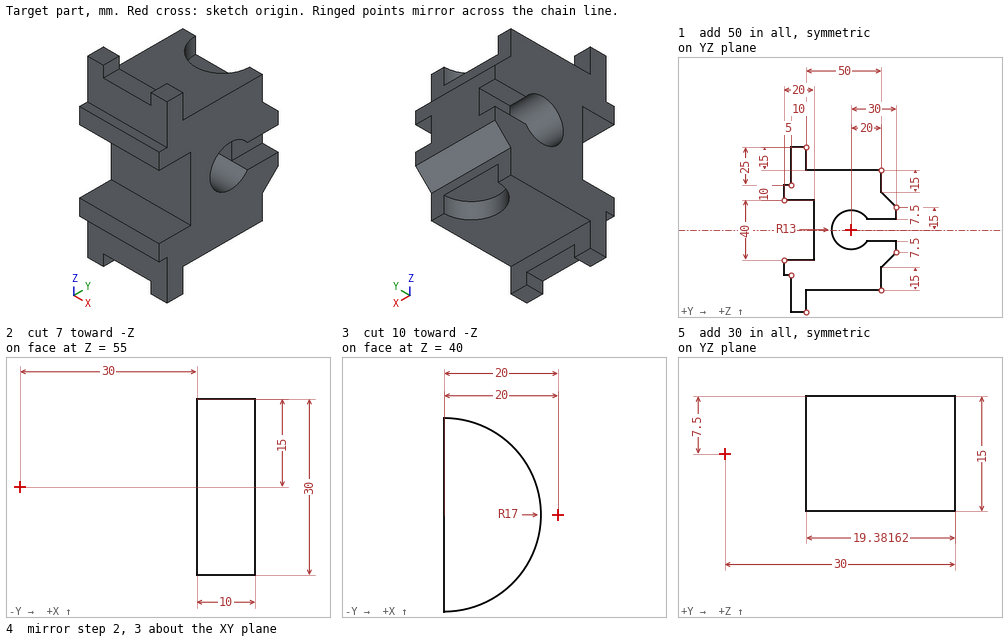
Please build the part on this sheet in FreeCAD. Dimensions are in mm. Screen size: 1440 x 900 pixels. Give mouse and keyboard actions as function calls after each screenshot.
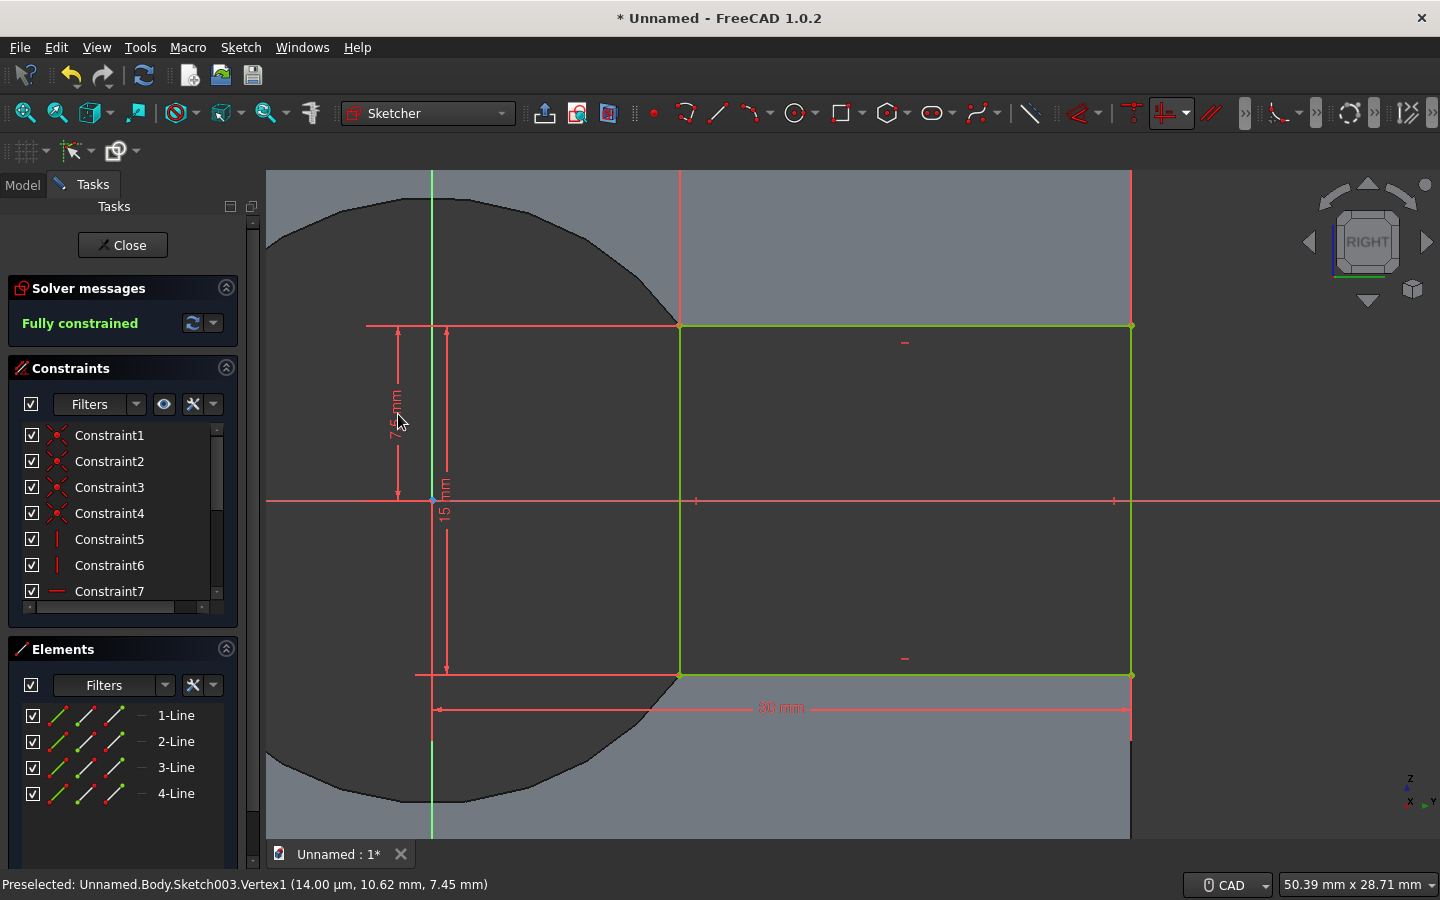
click(123, 245)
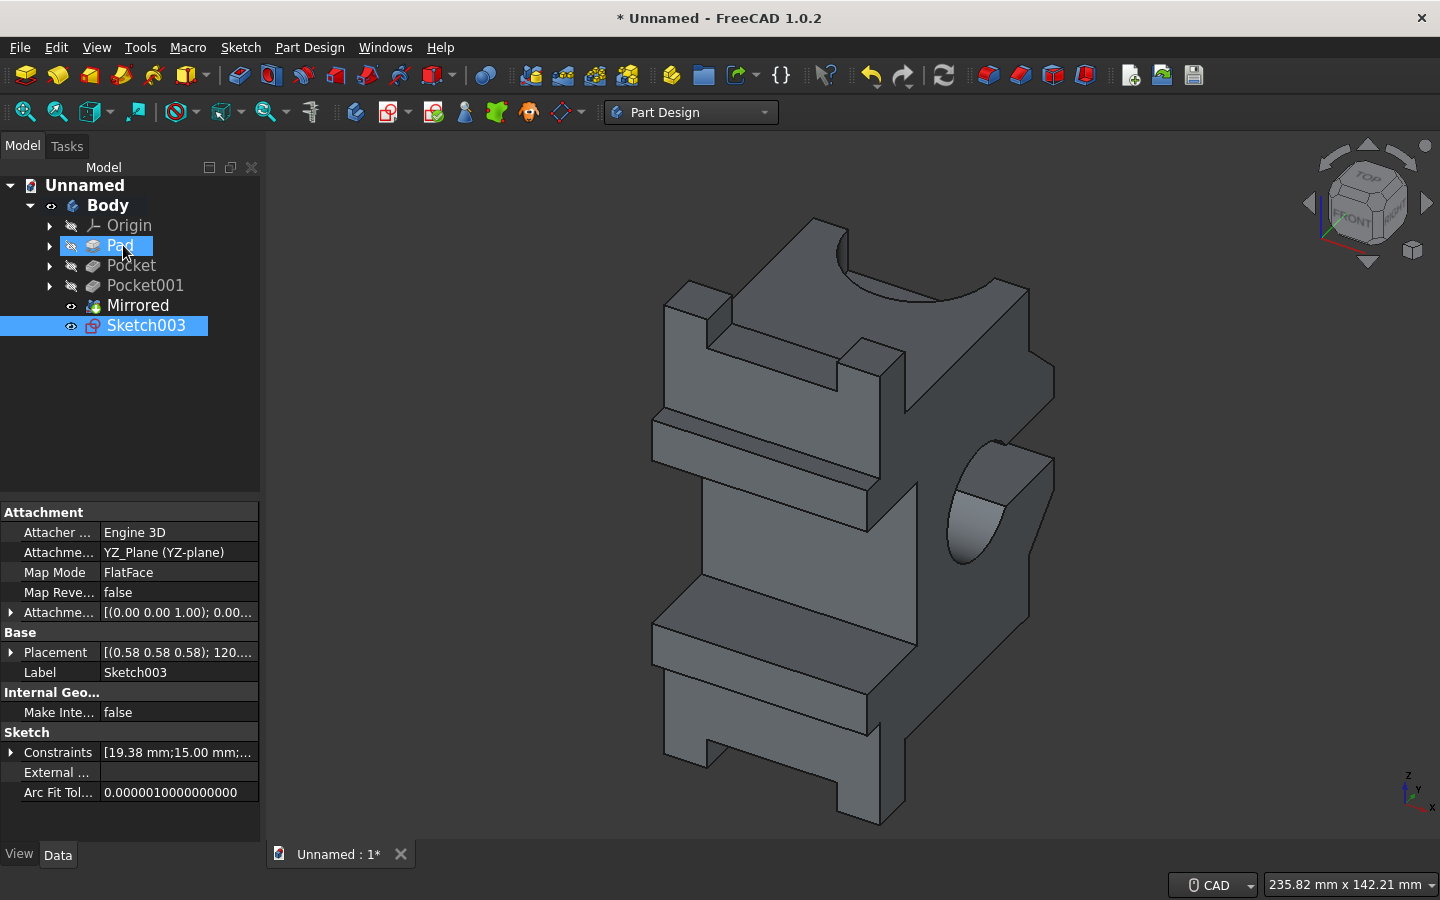
click(26, 76)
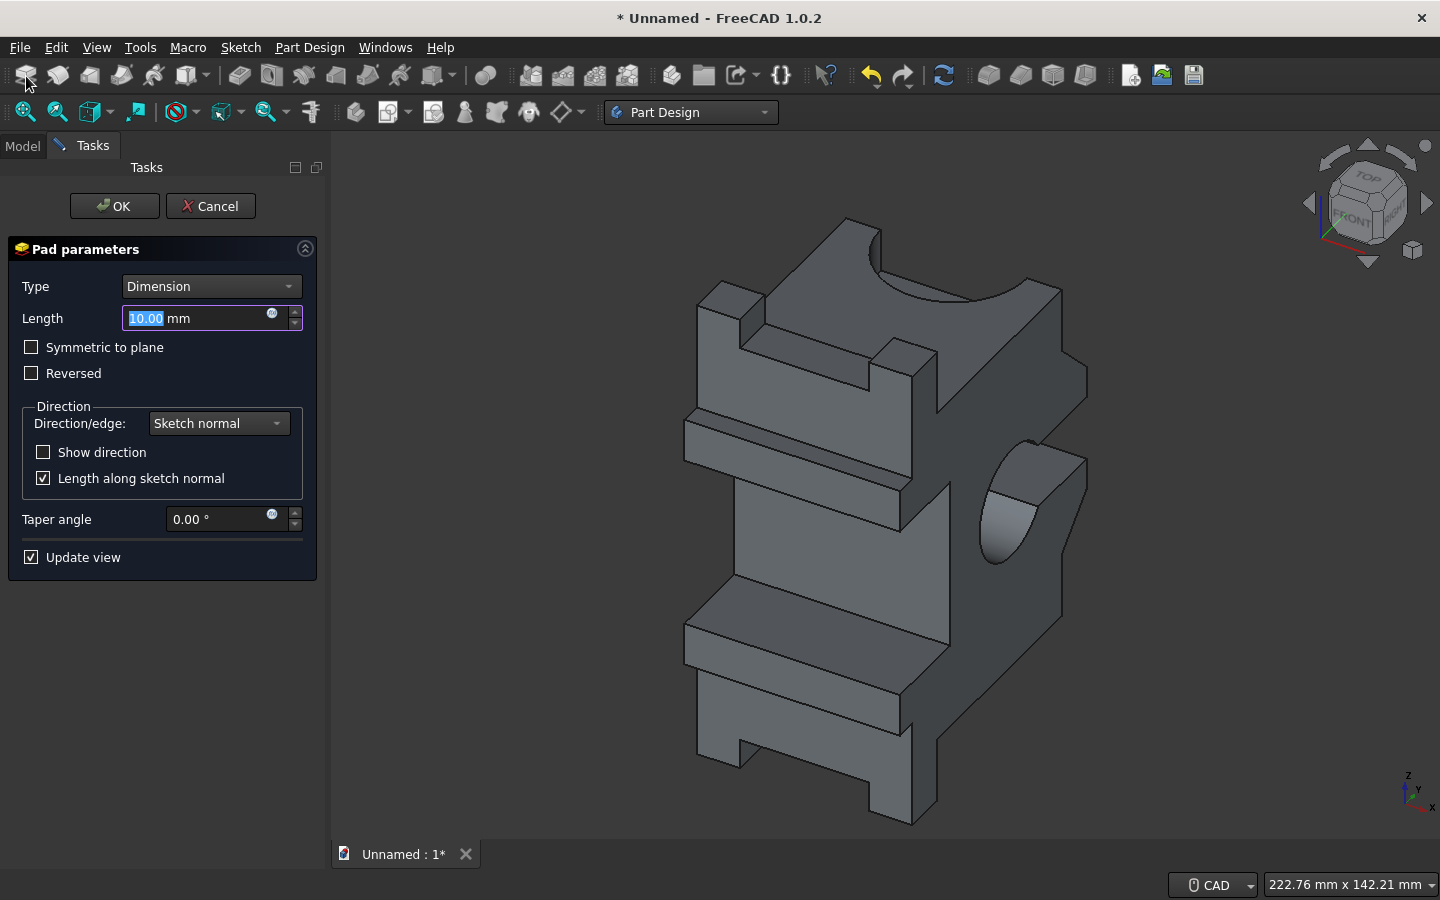
text(30)
key(Tab)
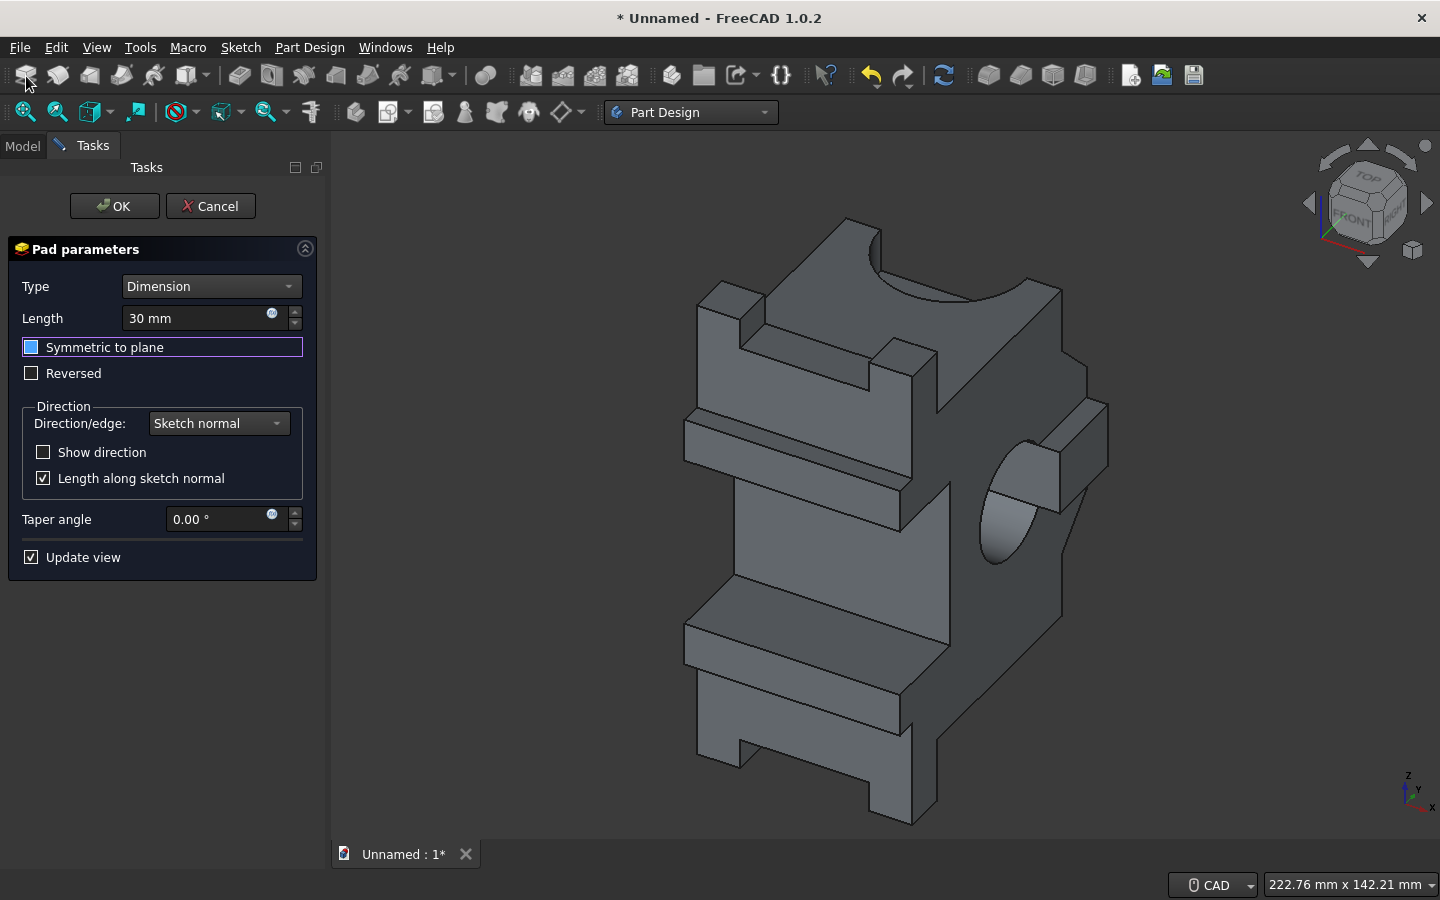
click(30, 347)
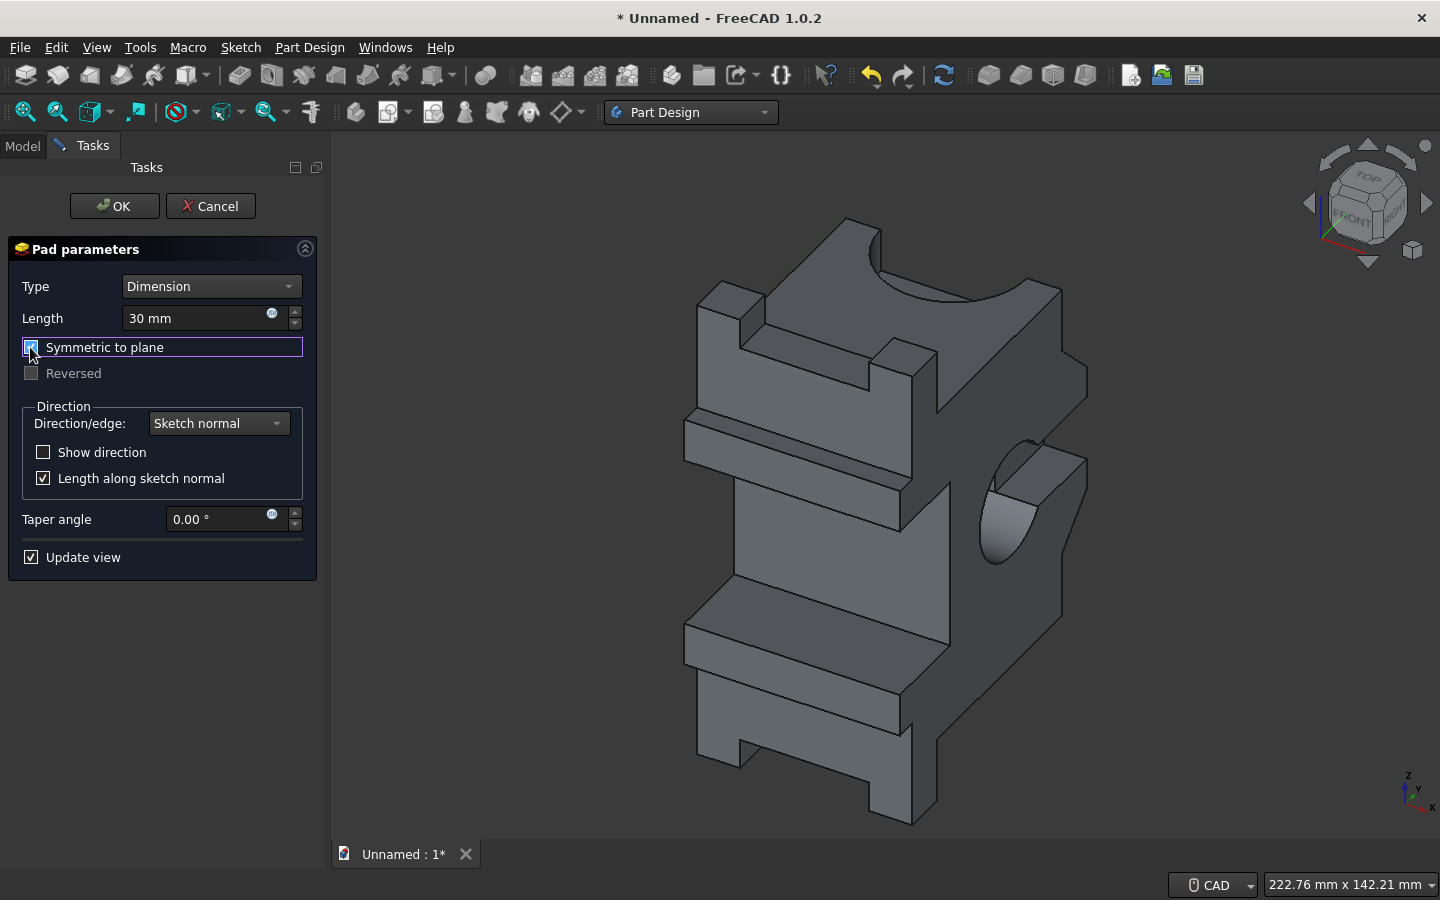
click(115, 206)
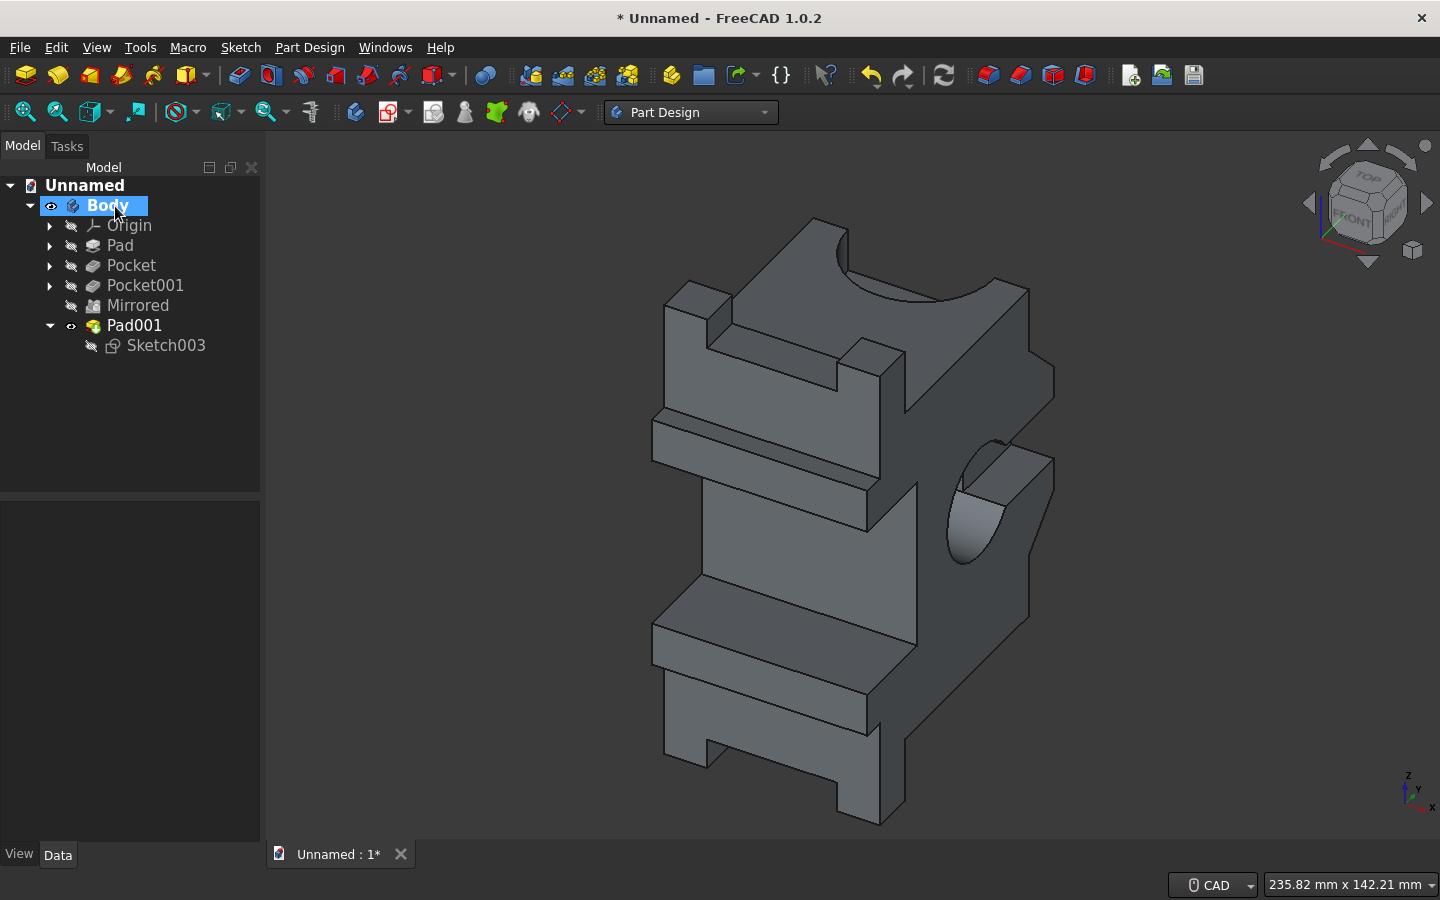
key(0)